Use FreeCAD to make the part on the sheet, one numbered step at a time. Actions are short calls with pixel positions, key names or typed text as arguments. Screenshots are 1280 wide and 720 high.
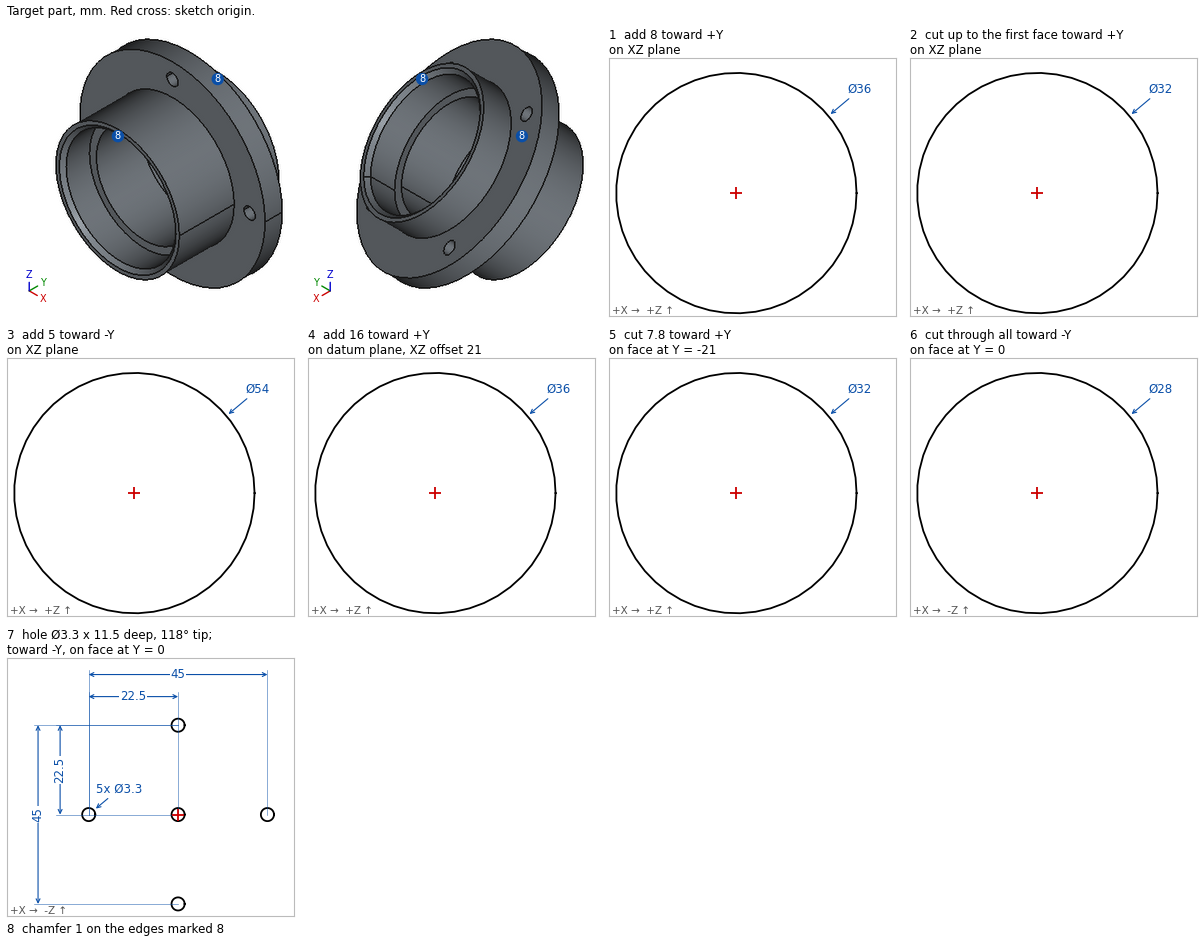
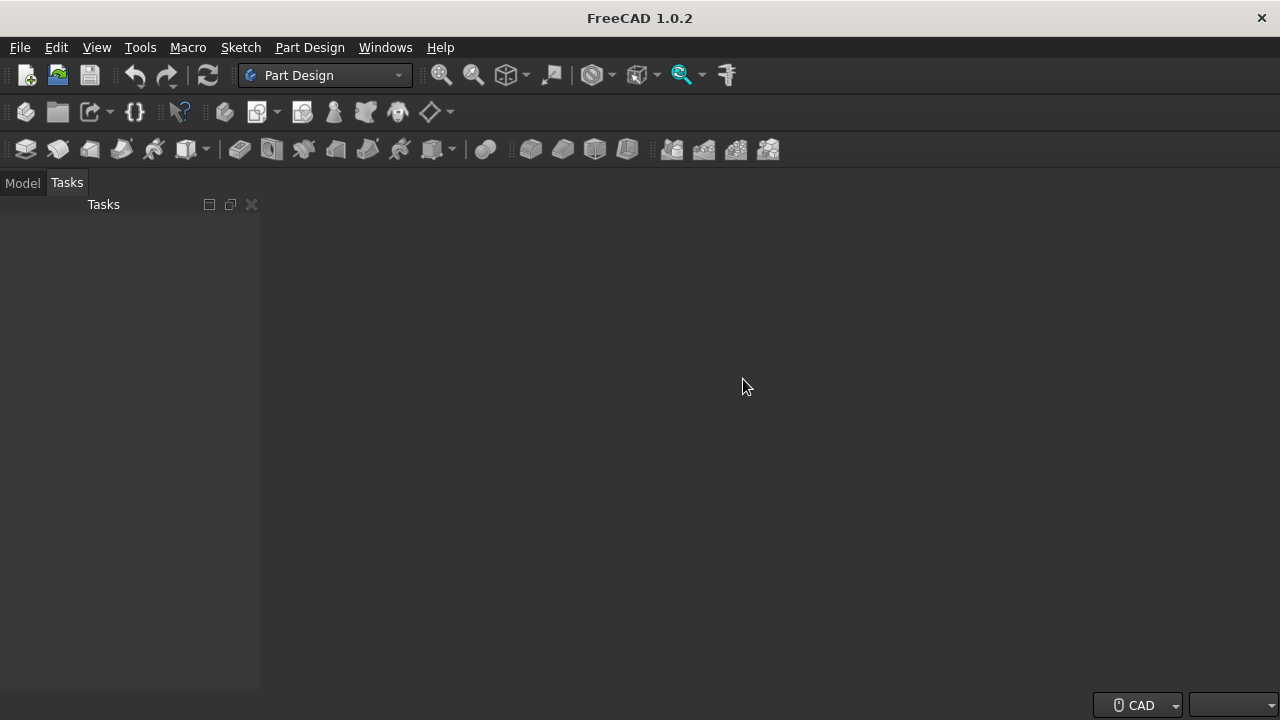
click(26, 76)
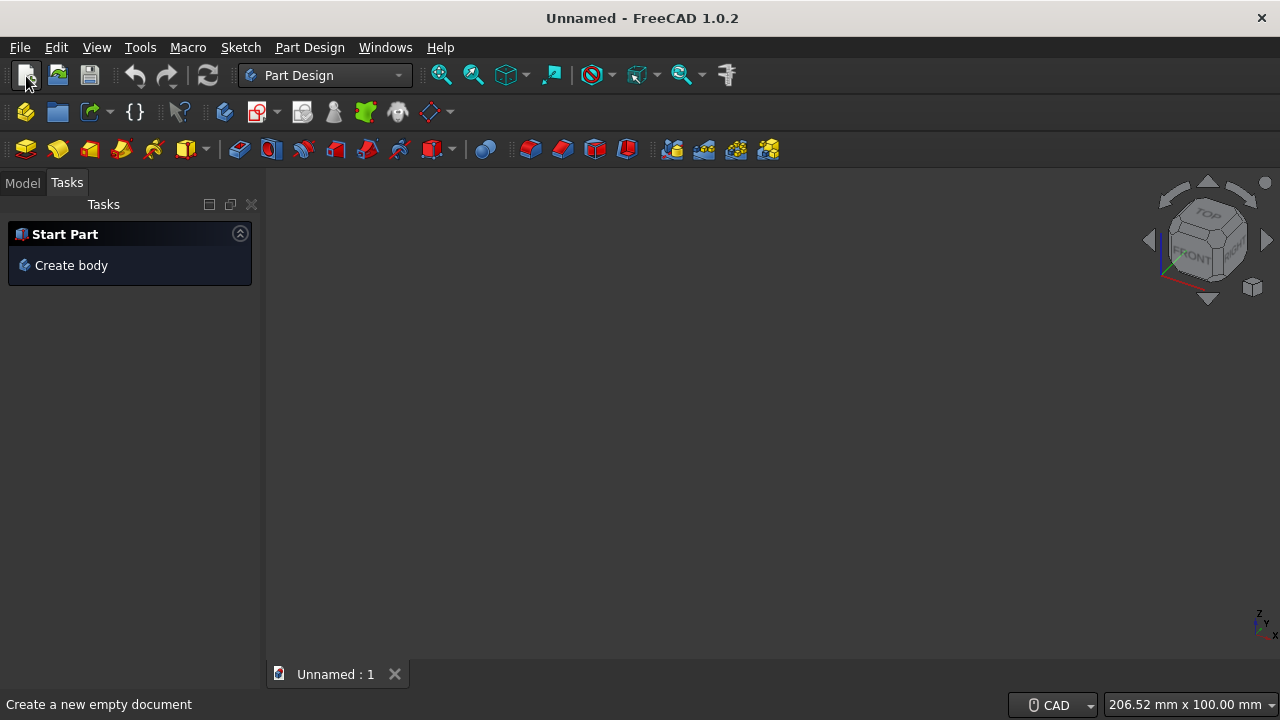
click(258, 112)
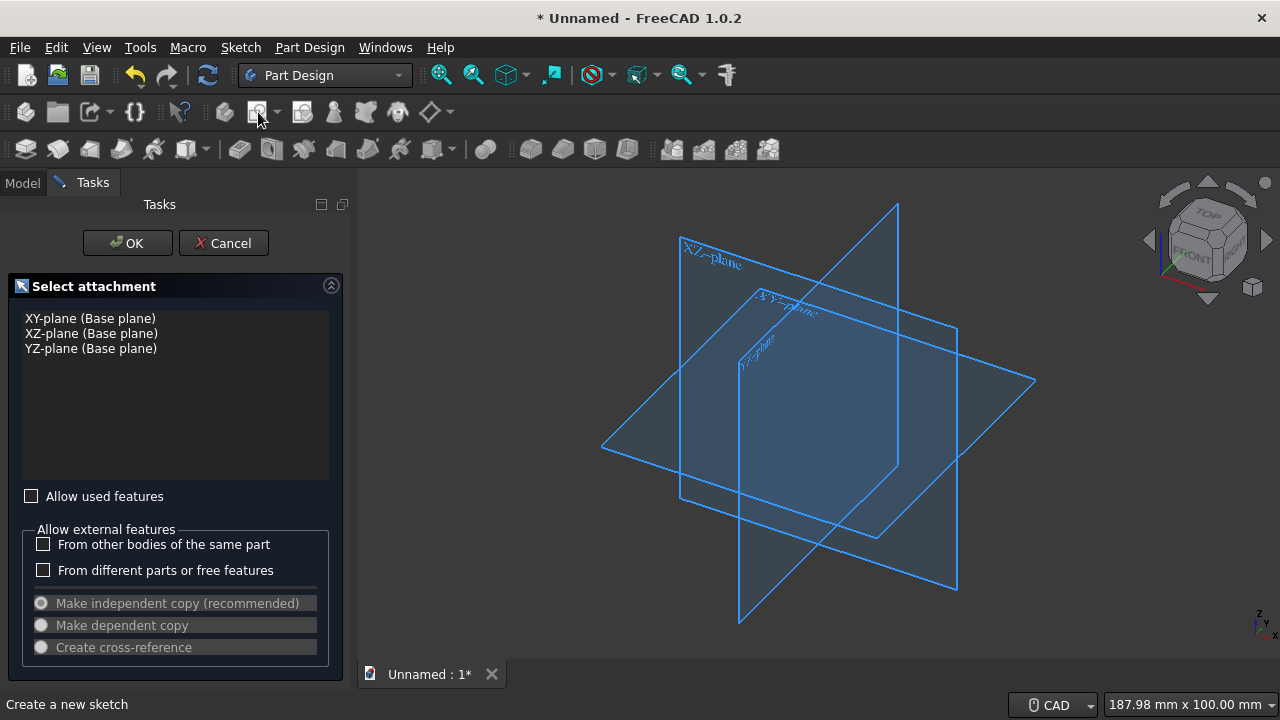
click(82, 334)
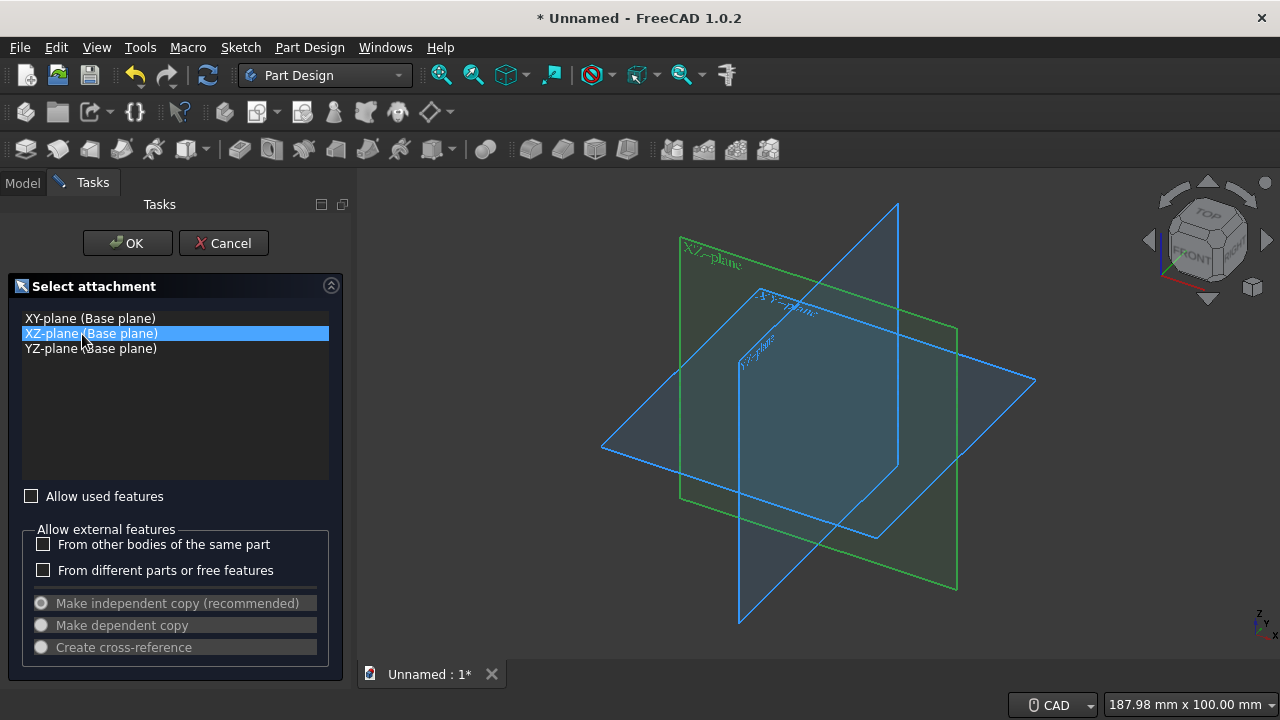
click(128, 243)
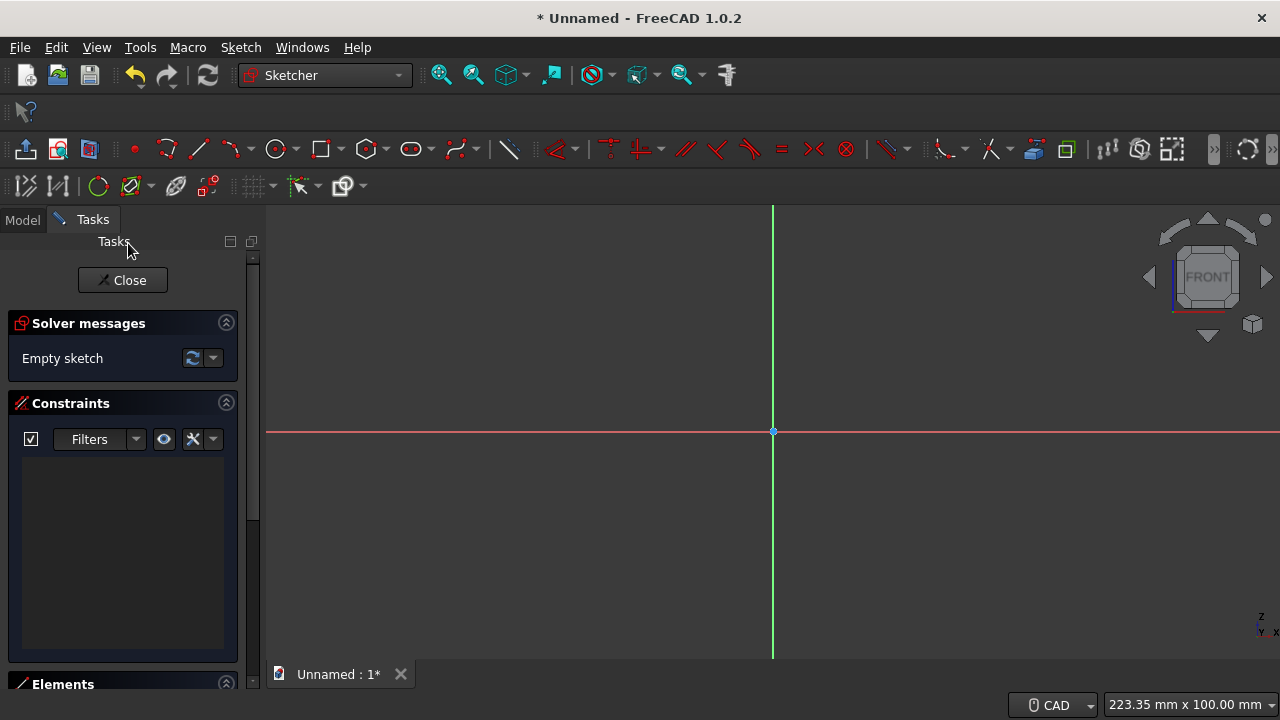
scroll(856, 432, up, 3)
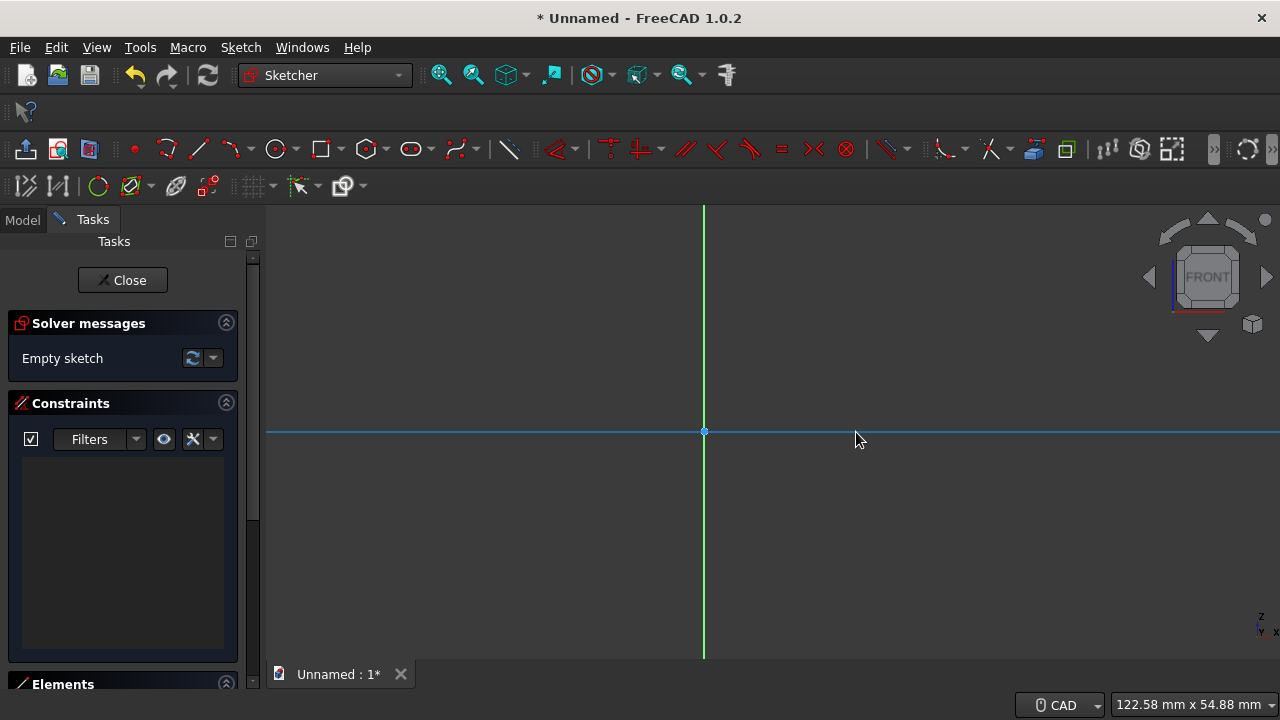
click(276, 150)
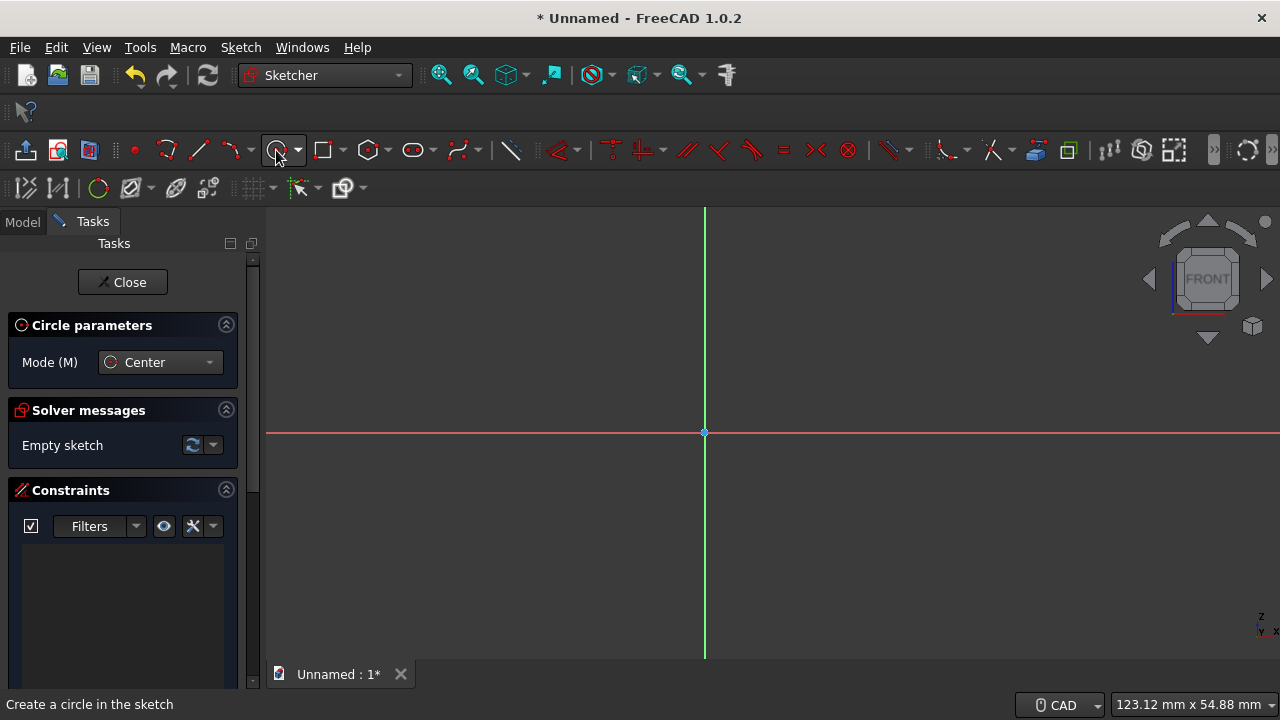
click(705, 433)
click(809, 328)
key(Escape)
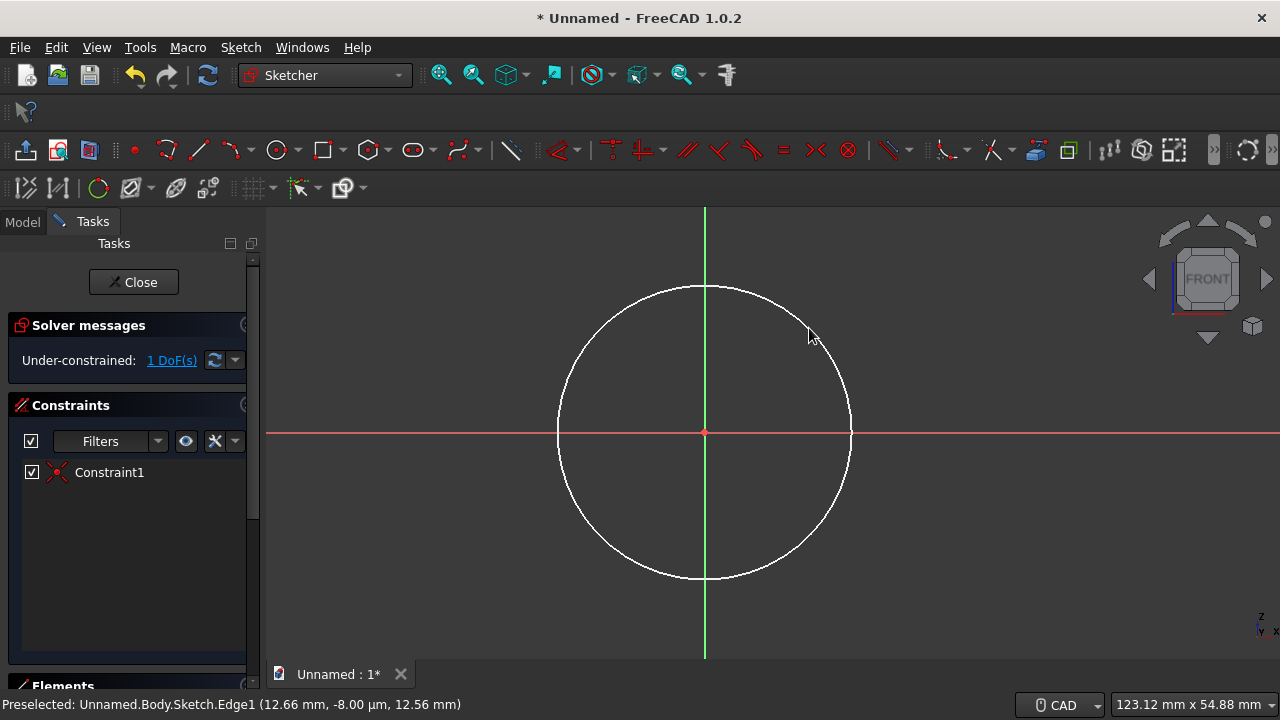
click(808, 328)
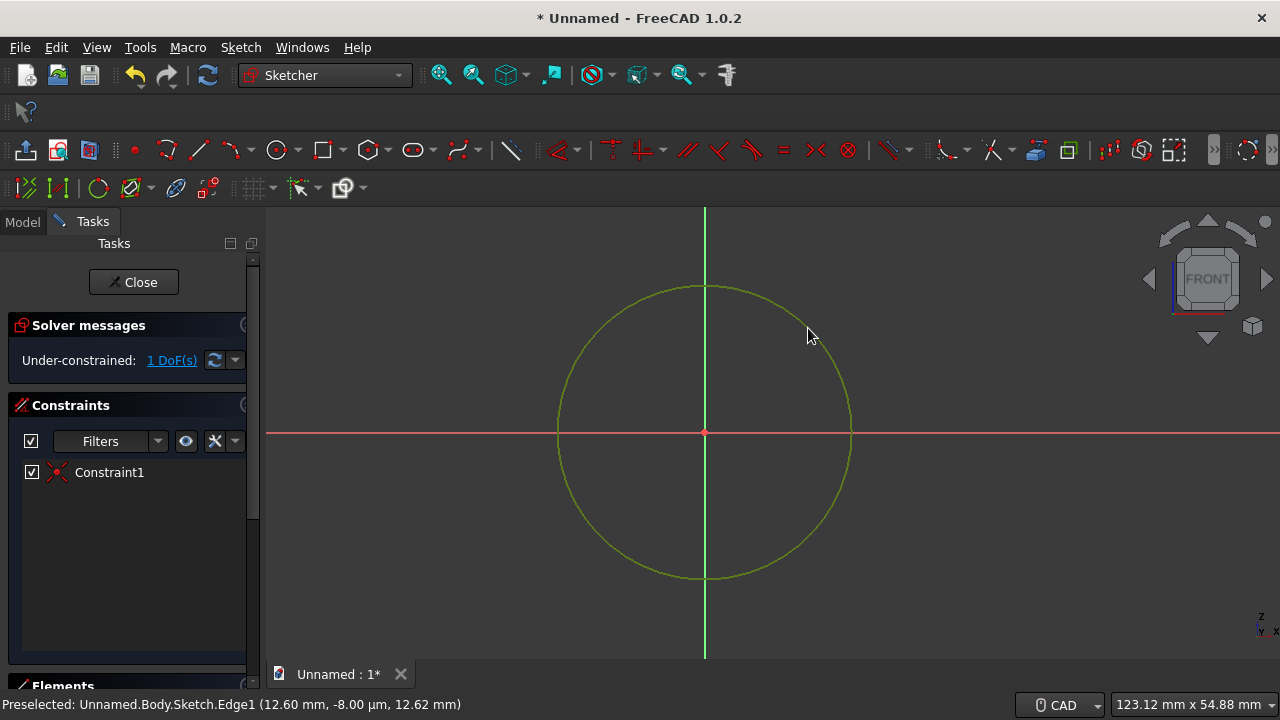
key(k)
key(o)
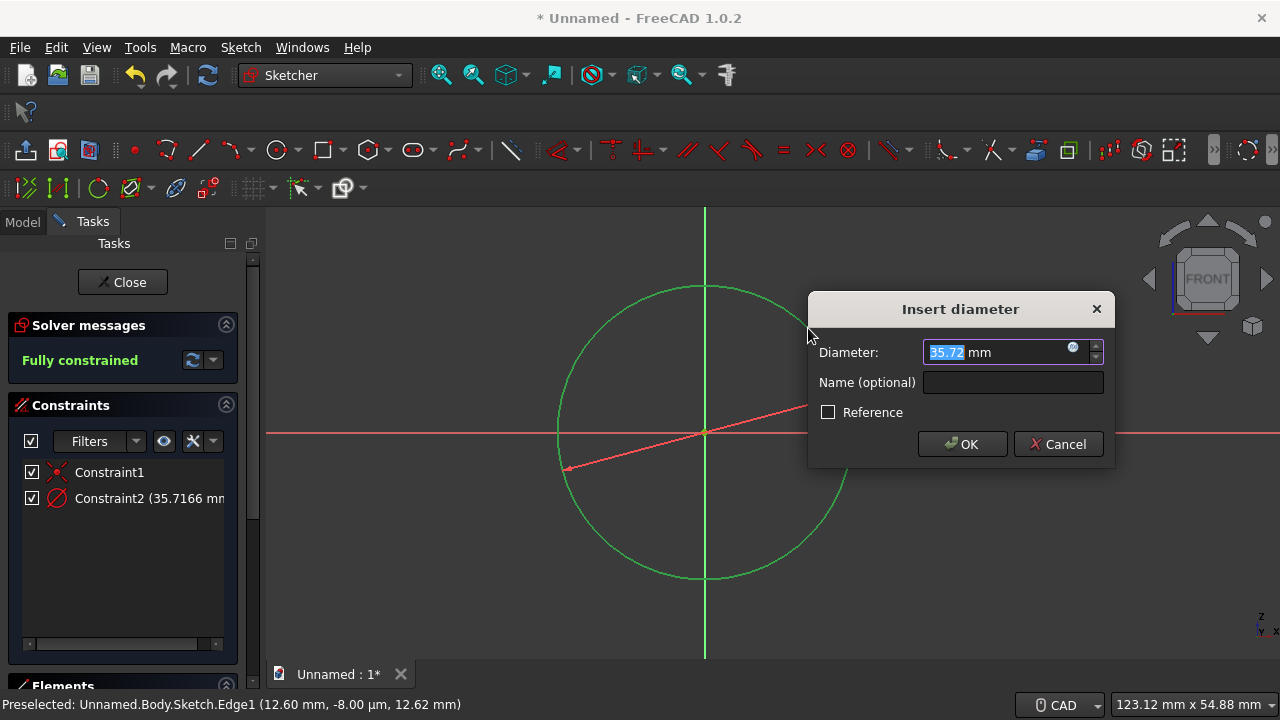
text(36)
key(Return)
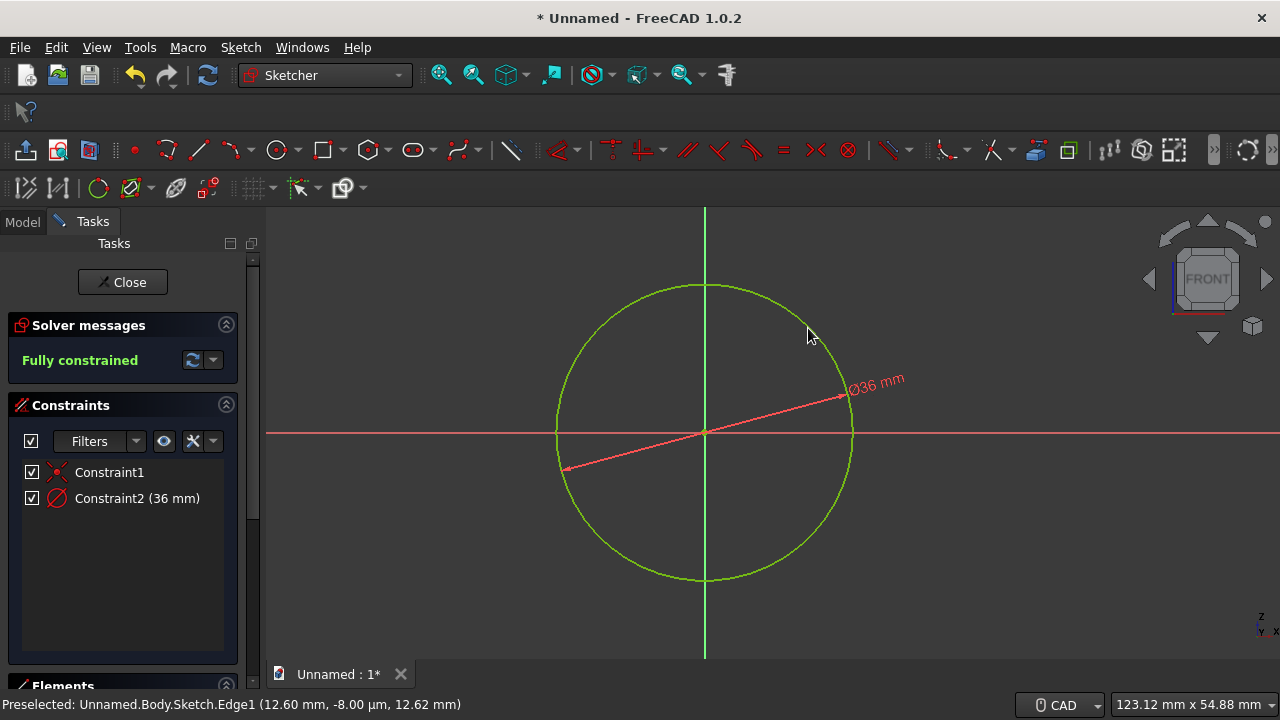
click(123, 282)